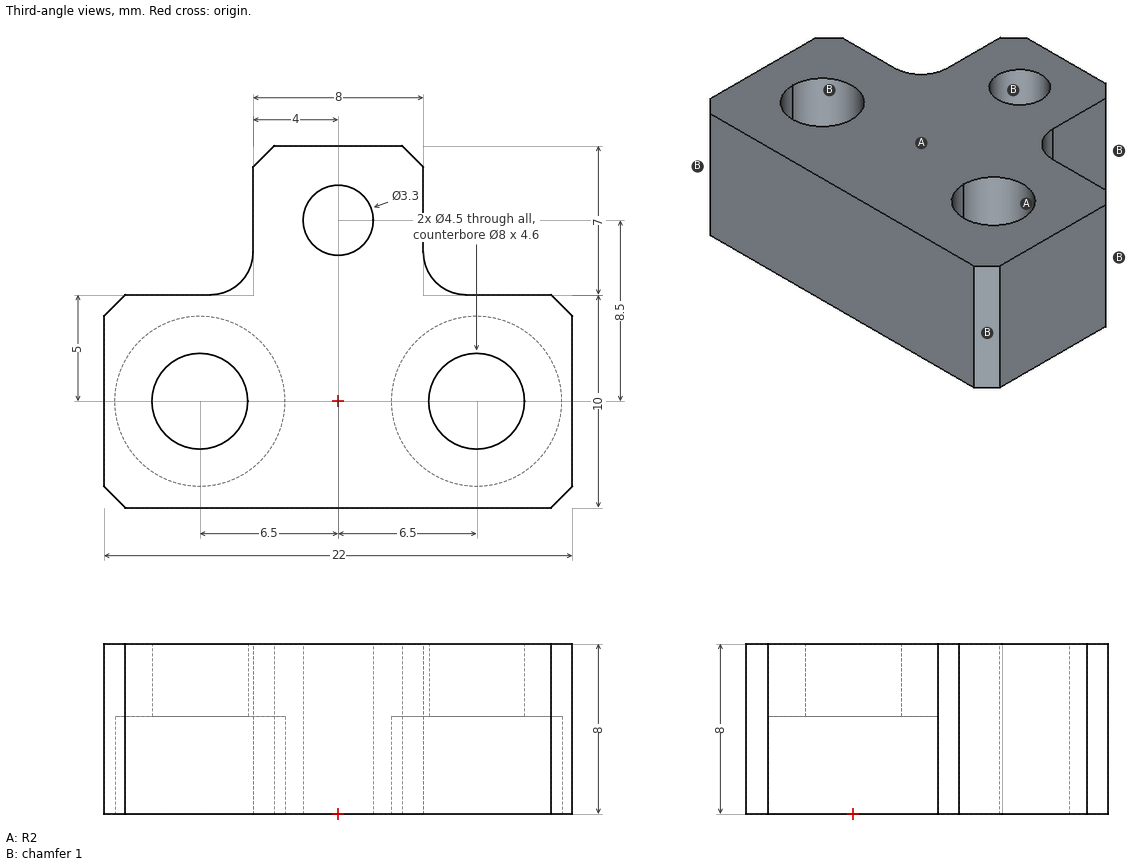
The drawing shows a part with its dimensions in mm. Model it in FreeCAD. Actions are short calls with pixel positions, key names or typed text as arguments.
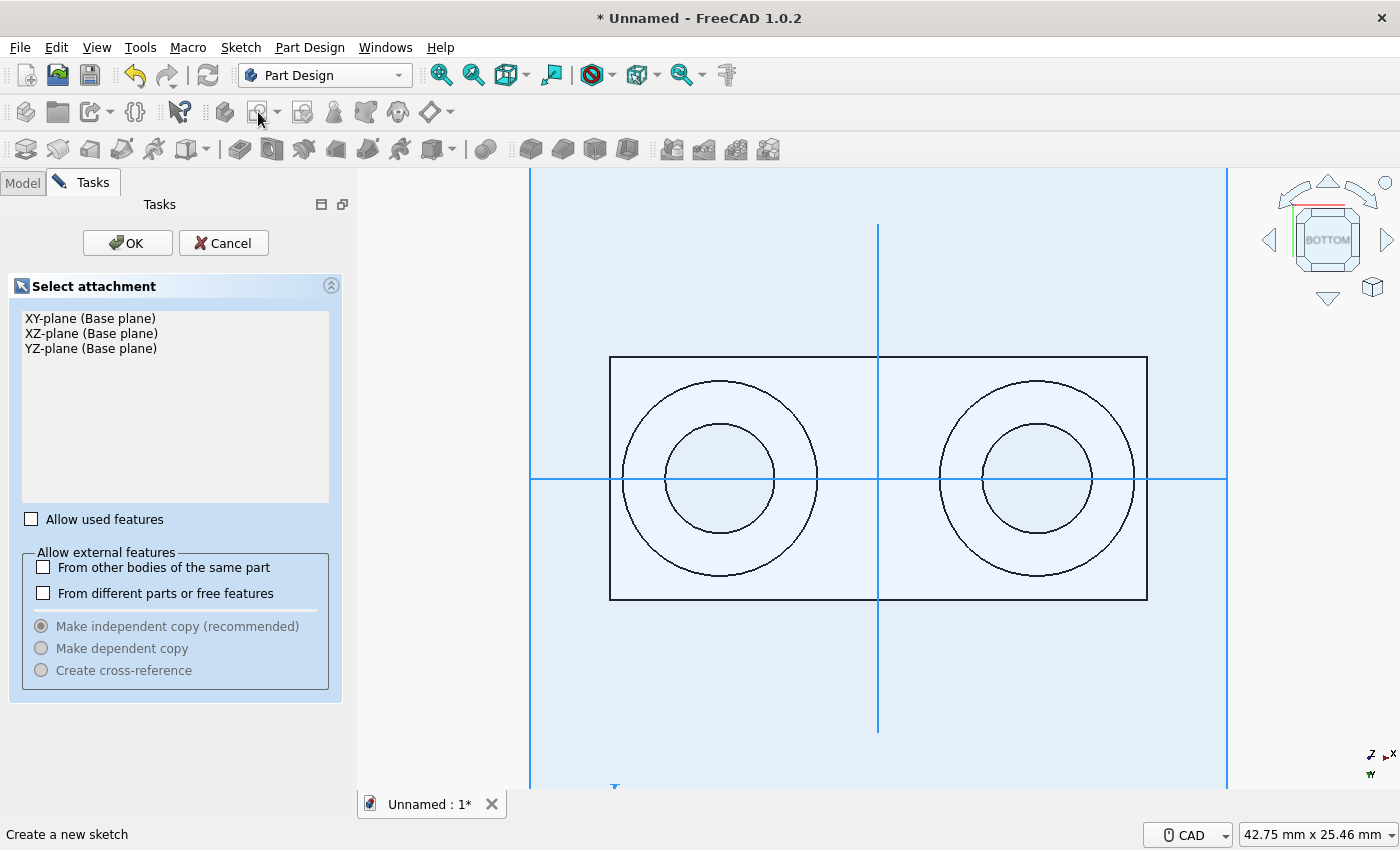
click(82, 318)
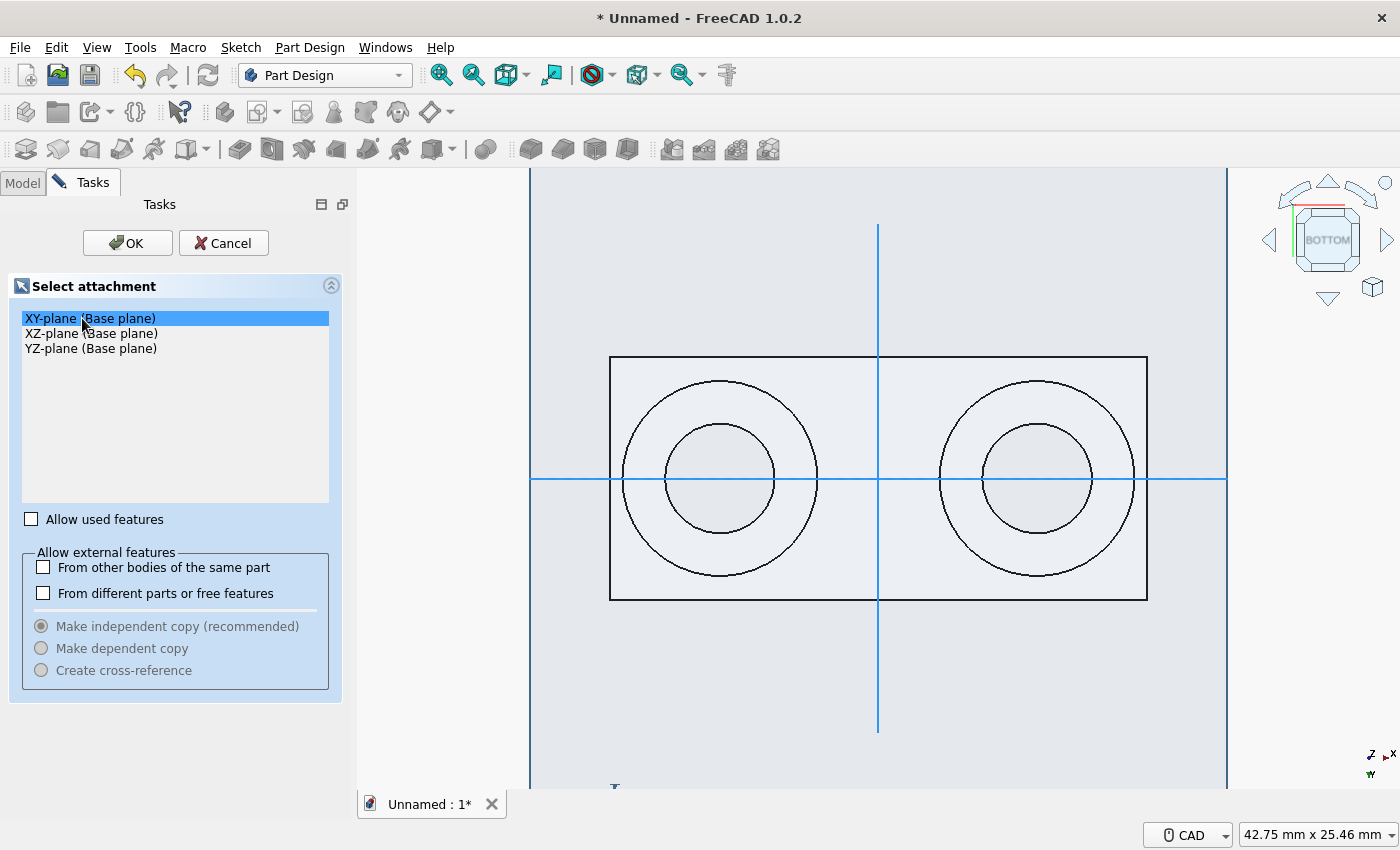
click(128, 243)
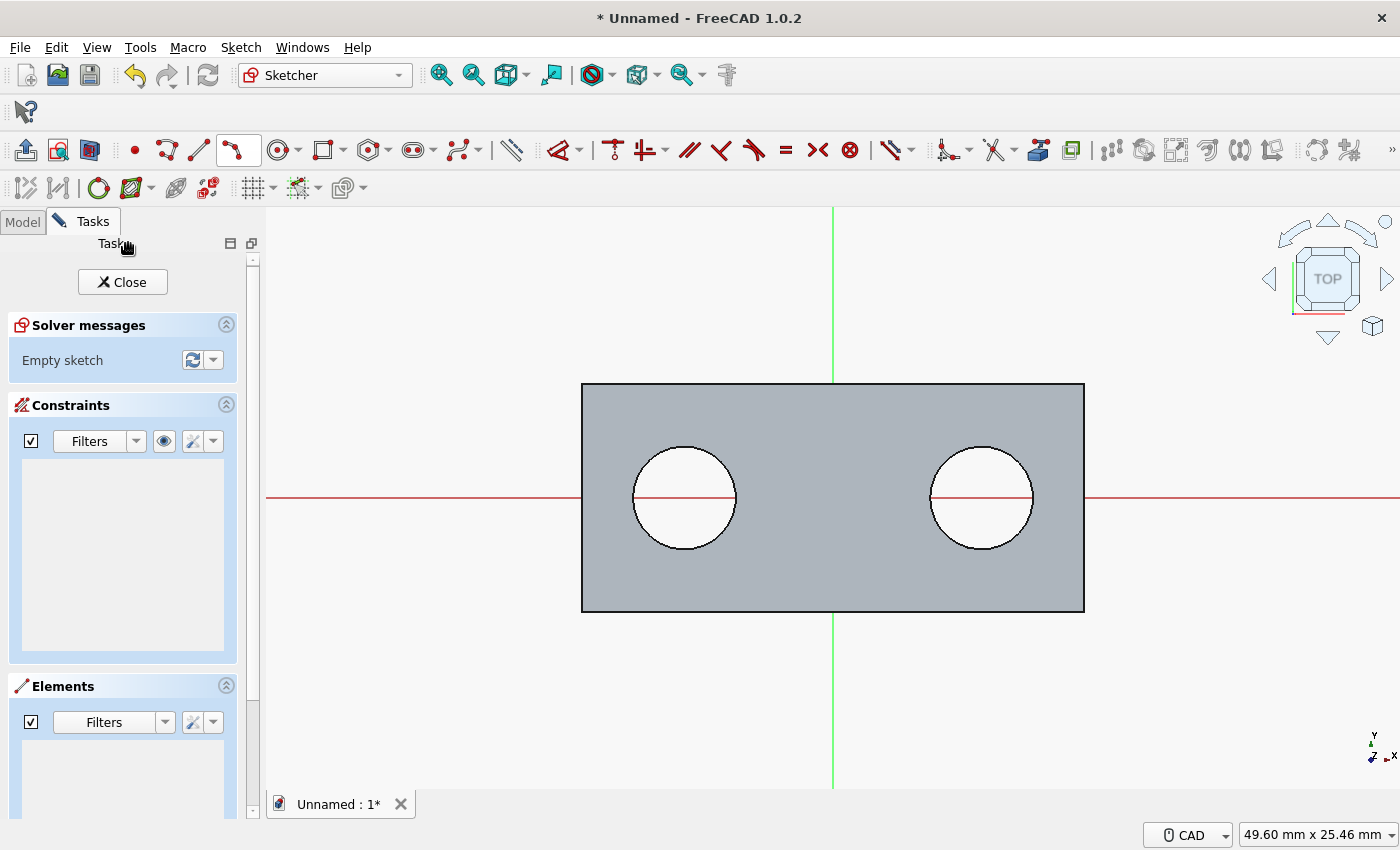
click(90, 150)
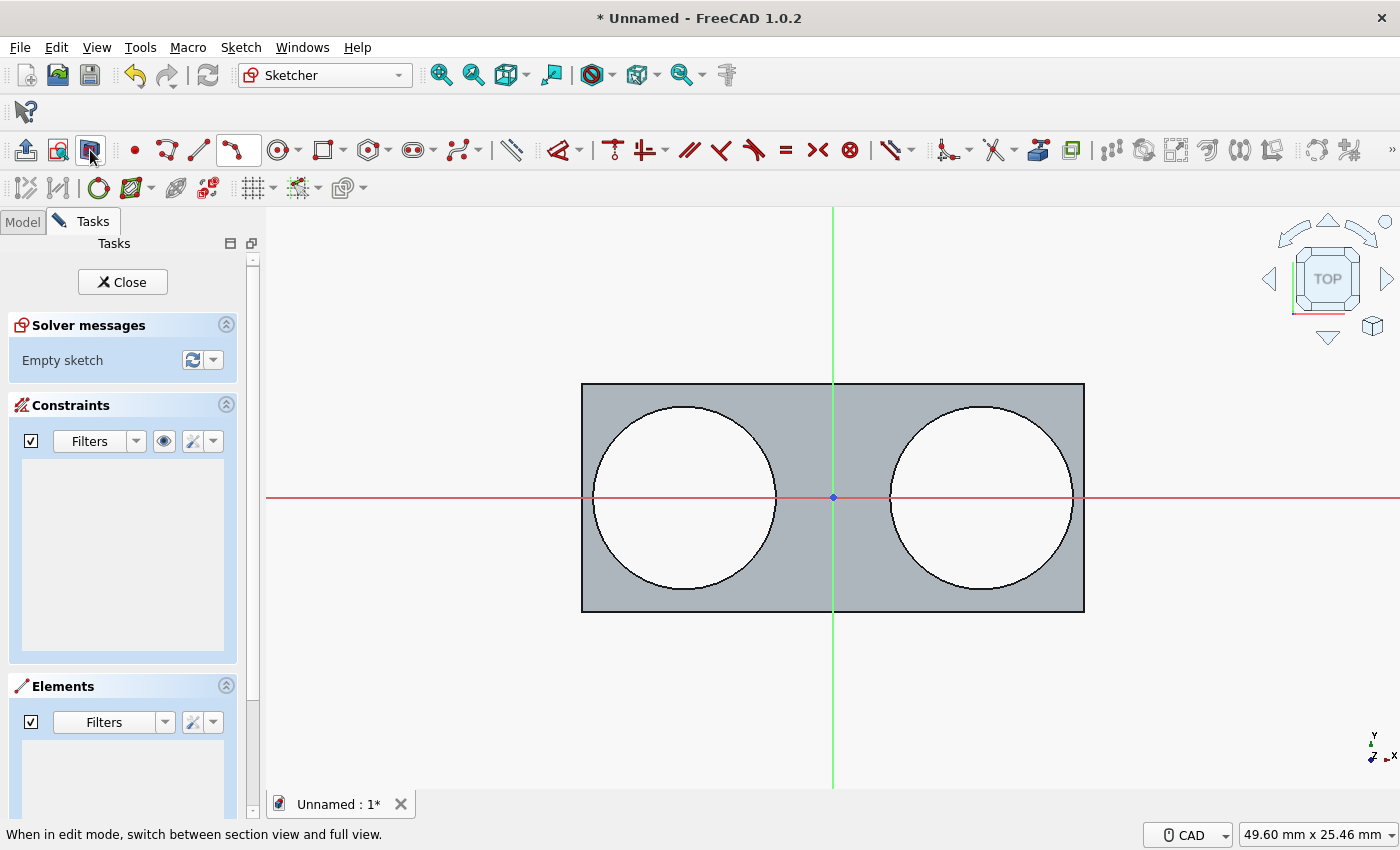
scroll(455, 761, down, 1)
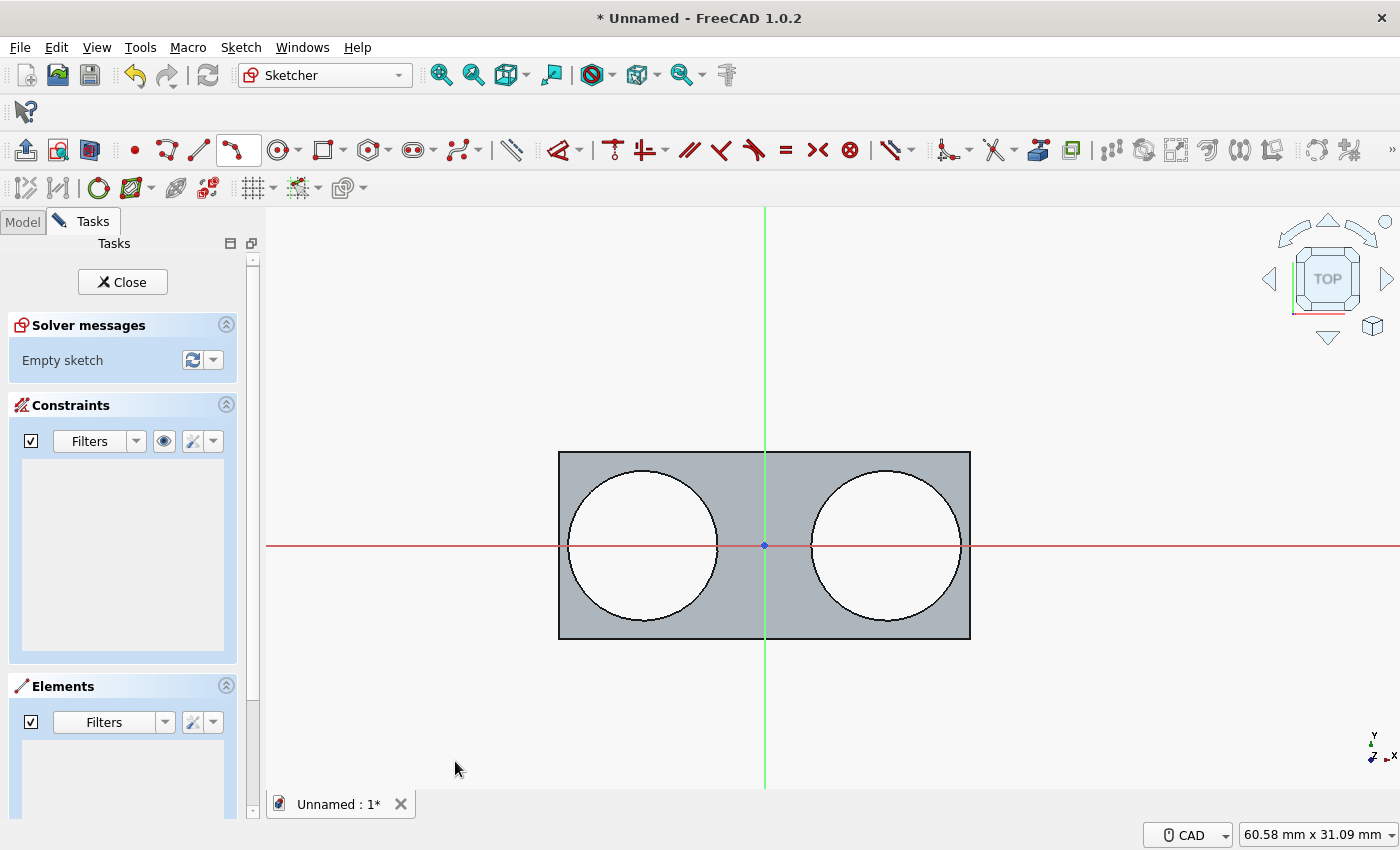
scroll(765, 355, up, 3)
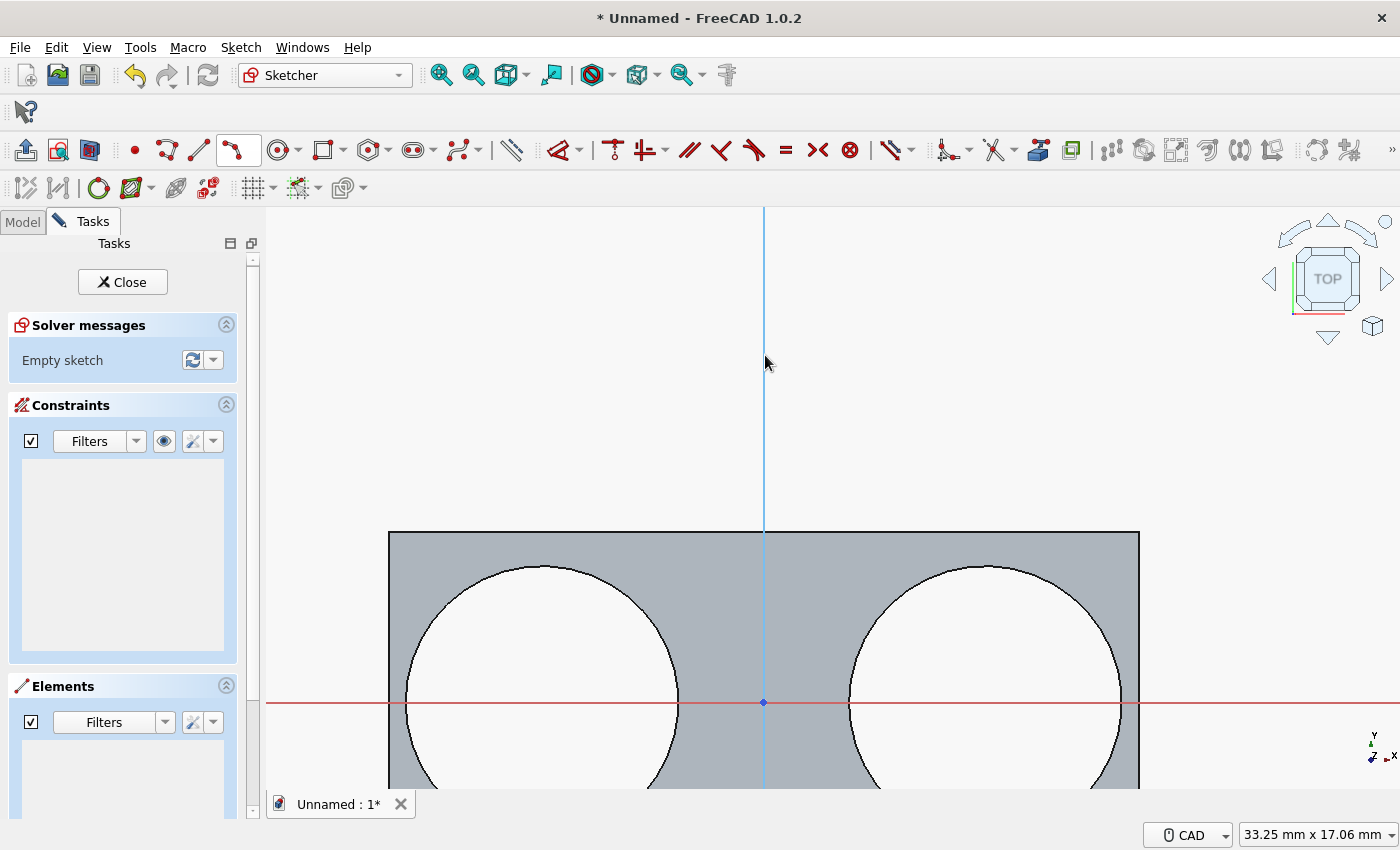
click(324, 150)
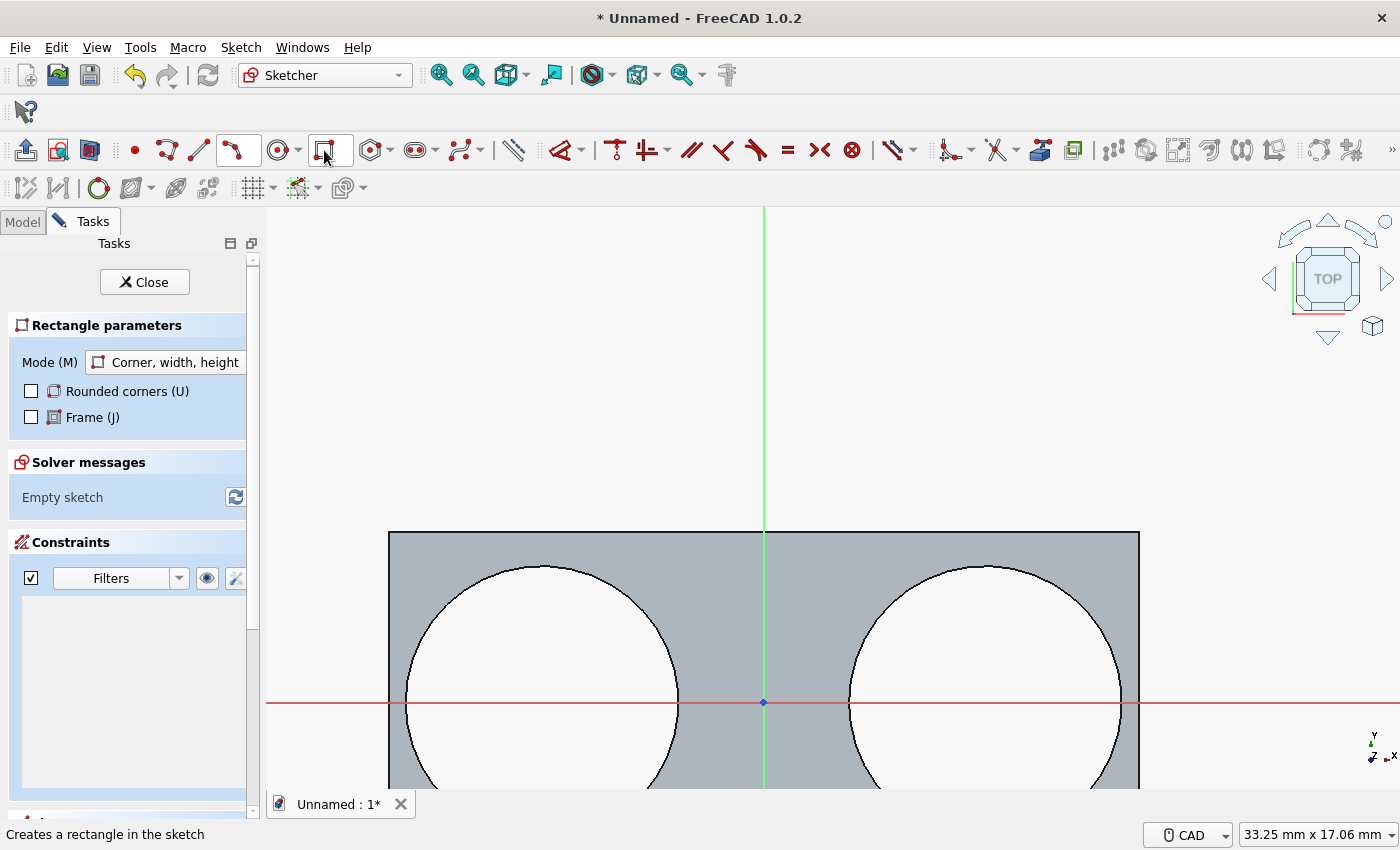
click(627, 293)
move(900, 532)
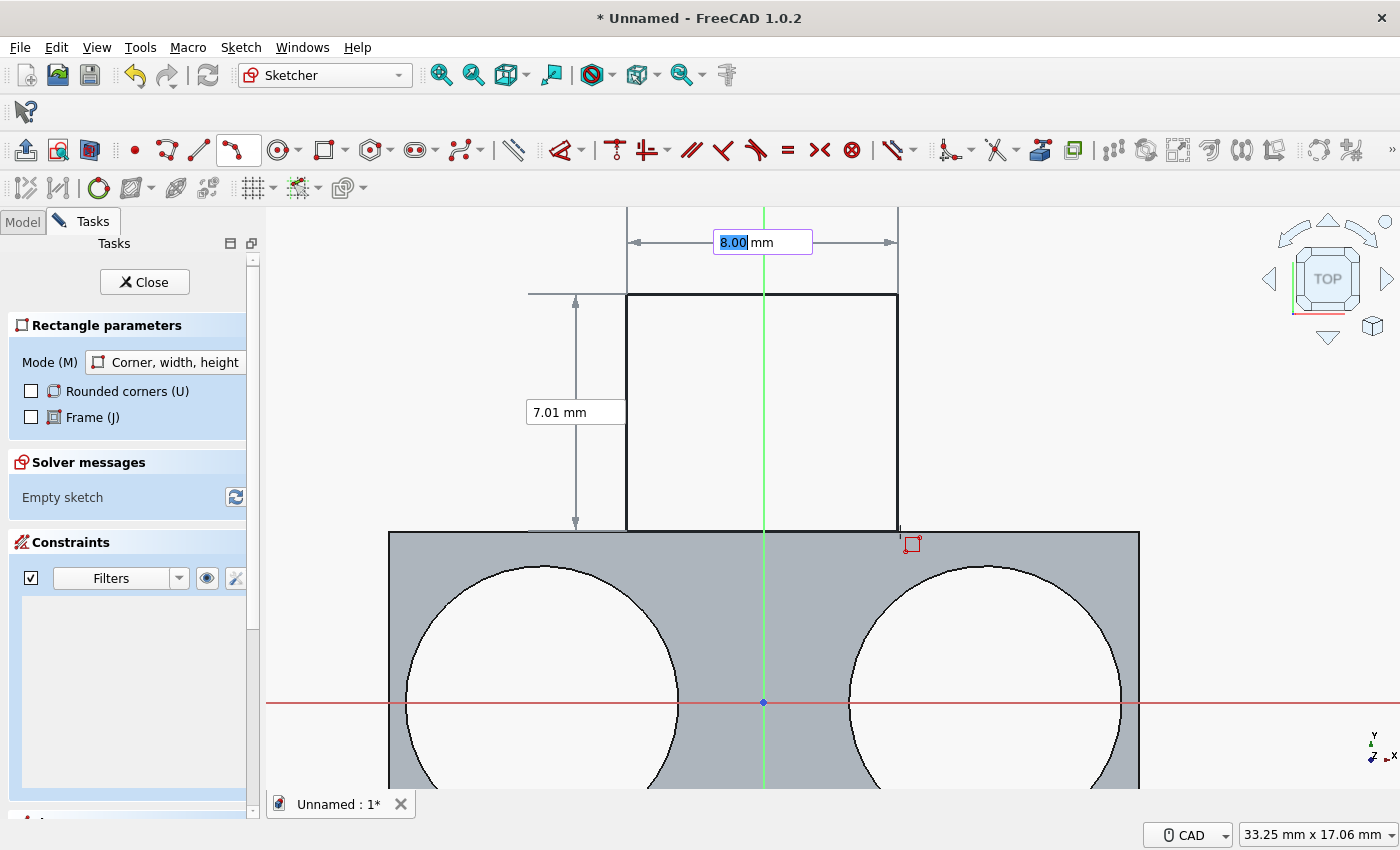
text(8)
key(Tab)
text(7)
key(Return)
key(Escape)